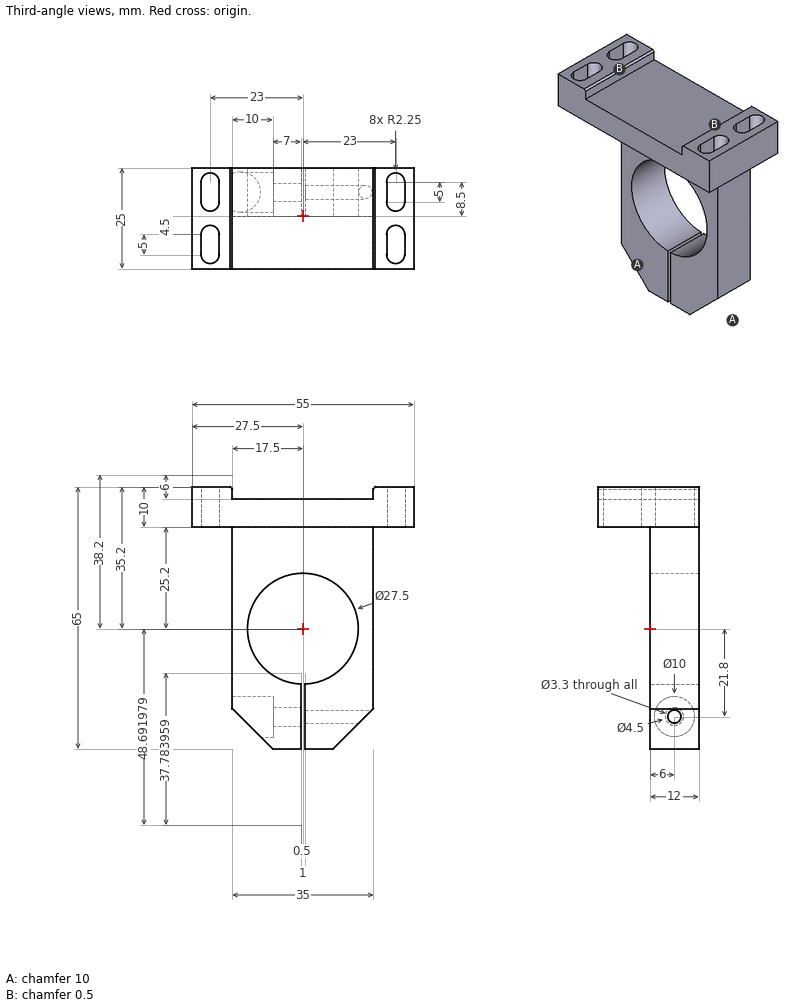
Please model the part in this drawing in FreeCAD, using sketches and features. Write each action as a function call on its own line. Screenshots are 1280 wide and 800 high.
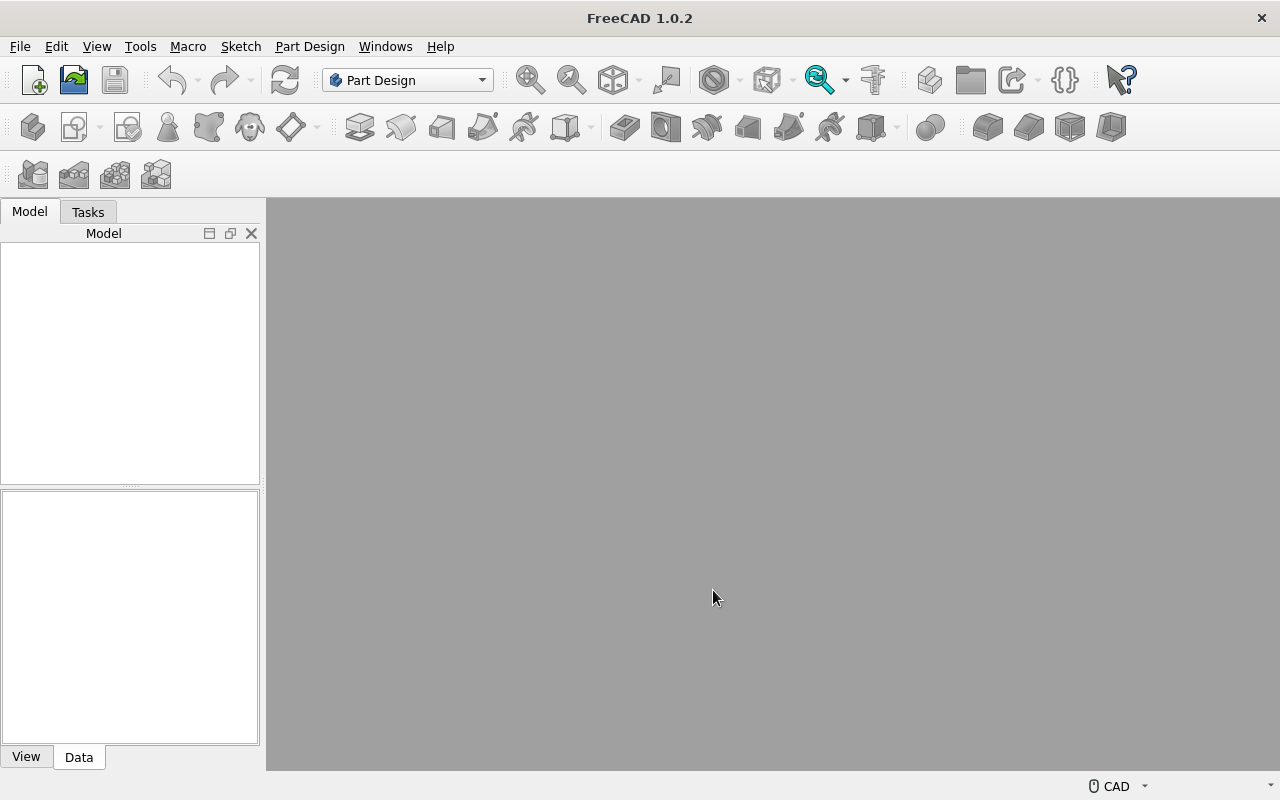
key(ctrl+n)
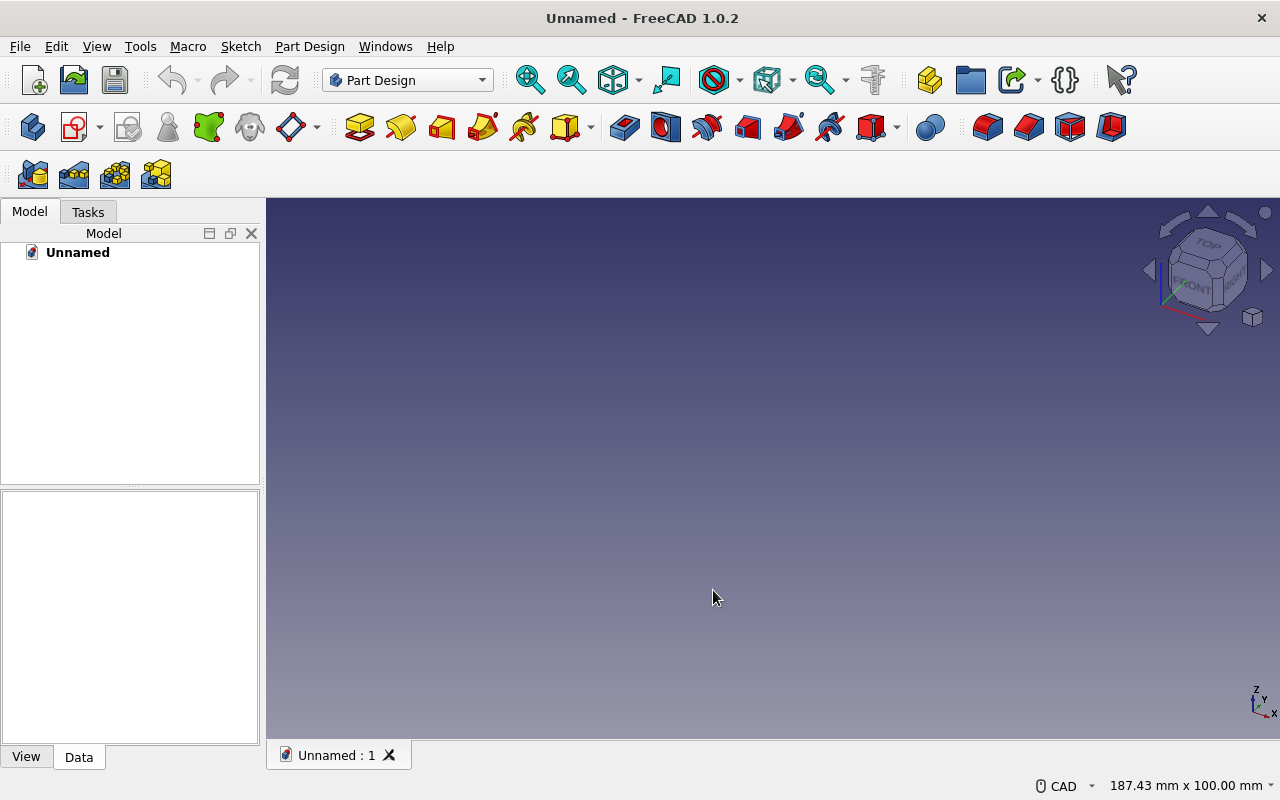
click(74, 128)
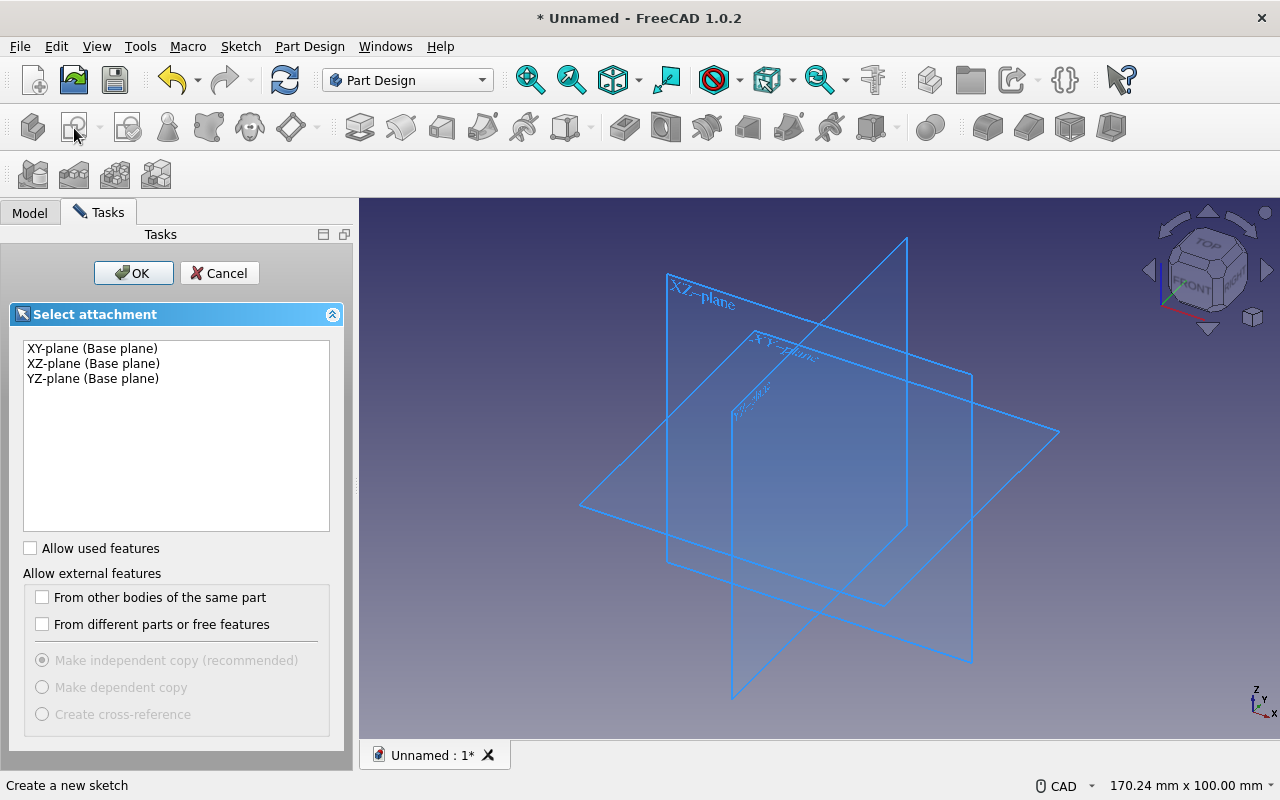
click(84, 364)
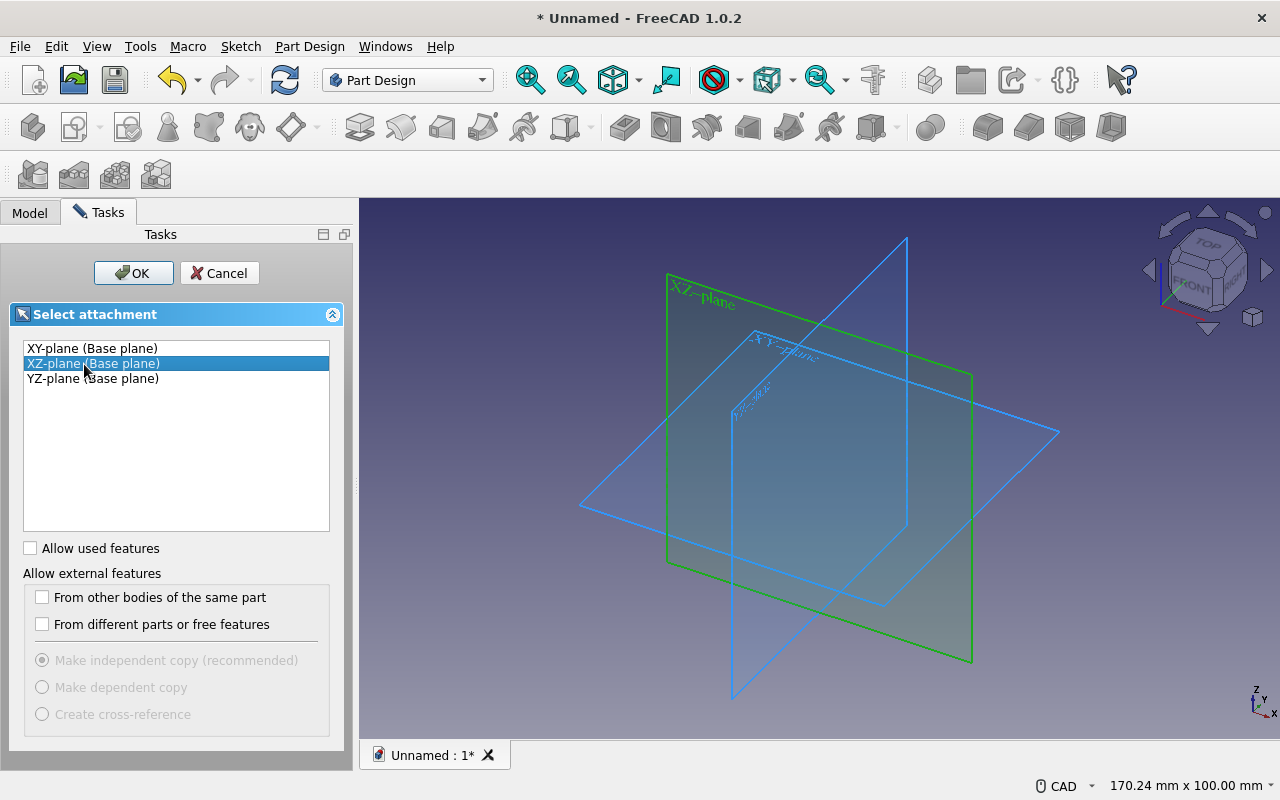
click(134, 273)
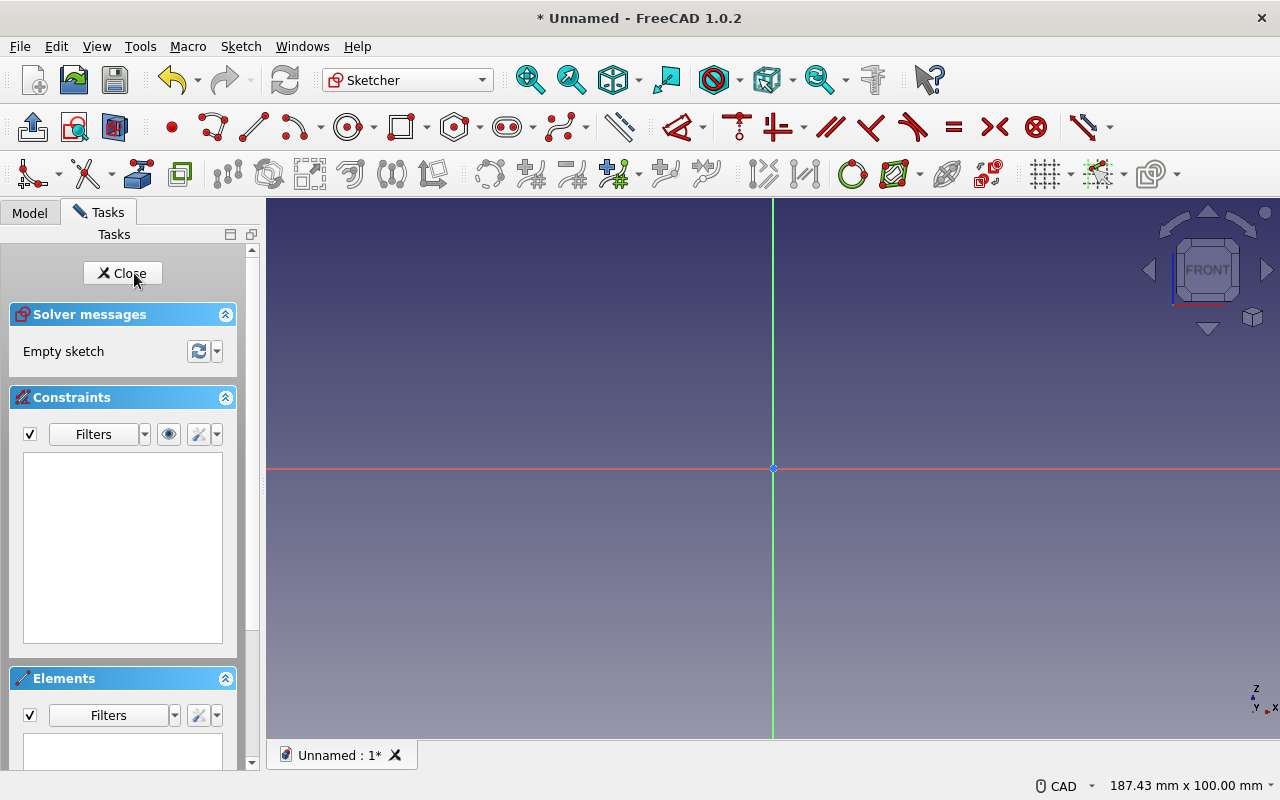
click(400, 128)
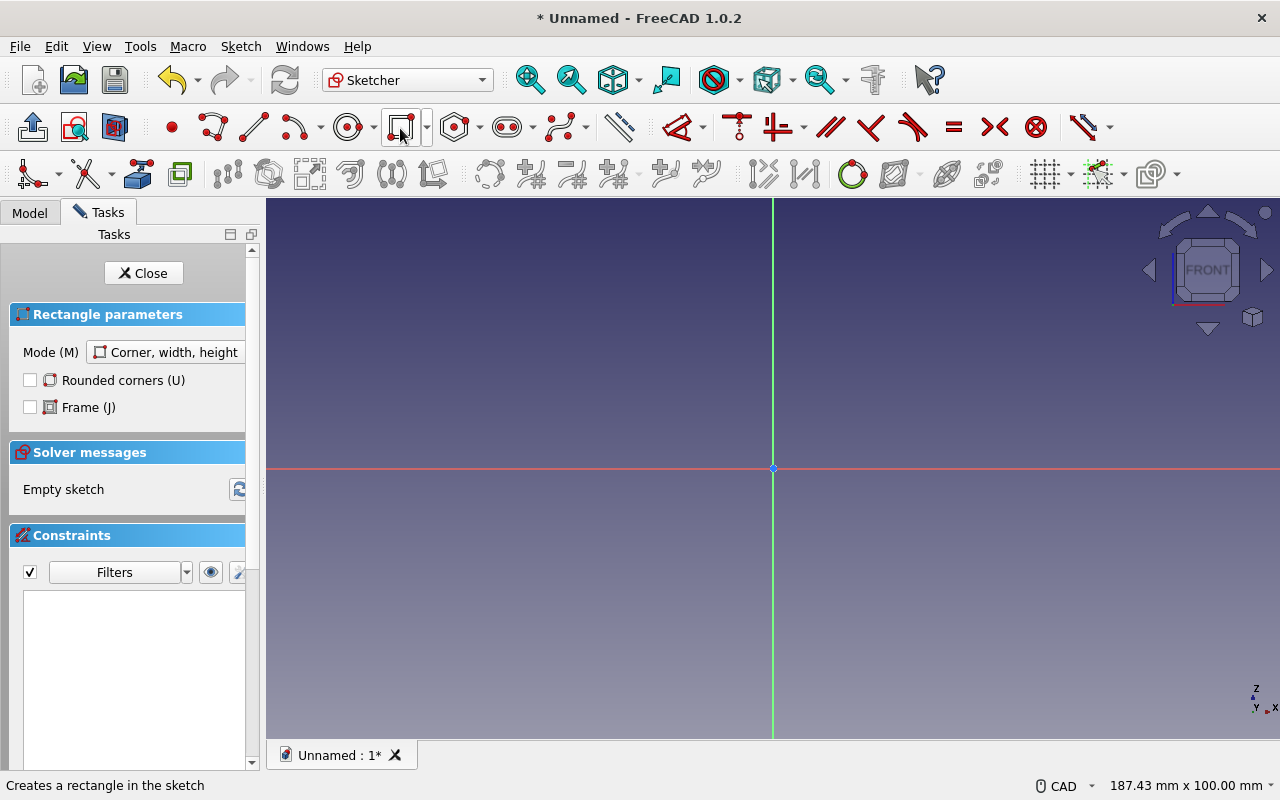
click(678, 278)
click(868, 630)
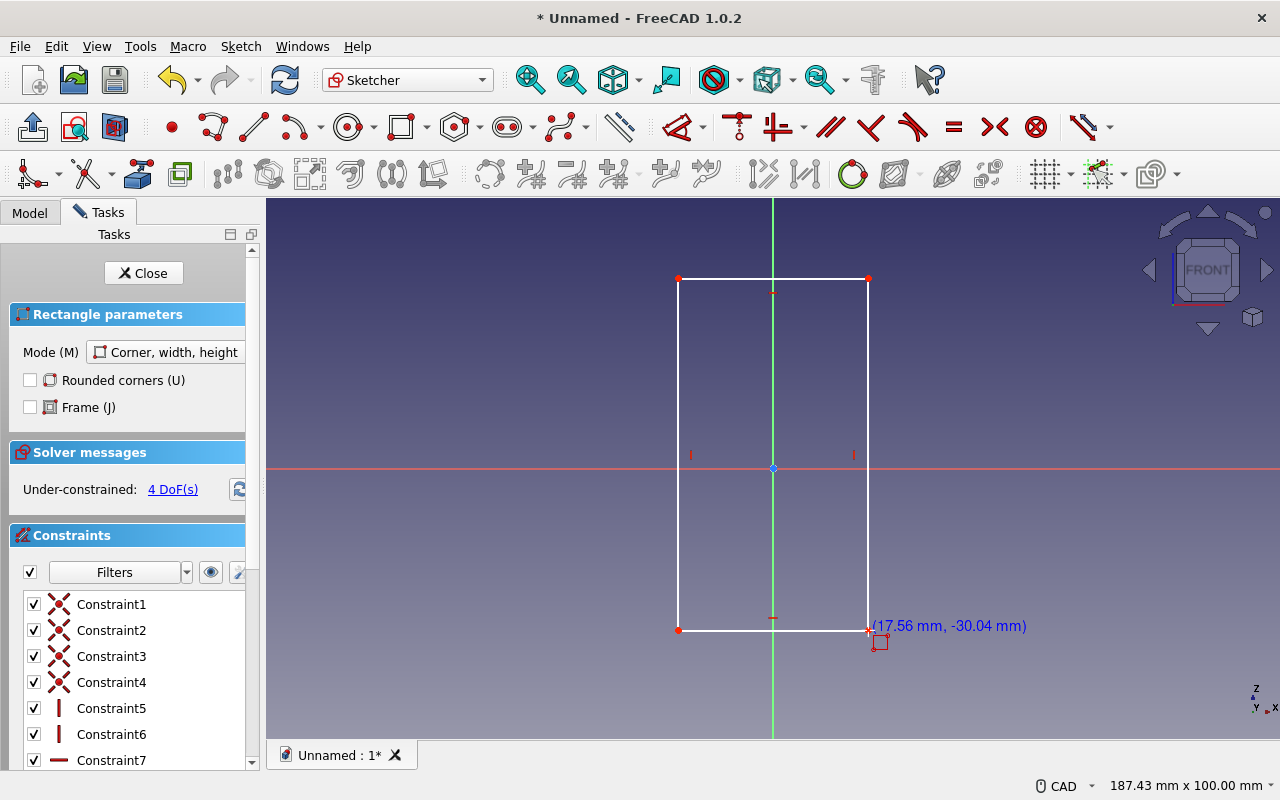
click(348, 128)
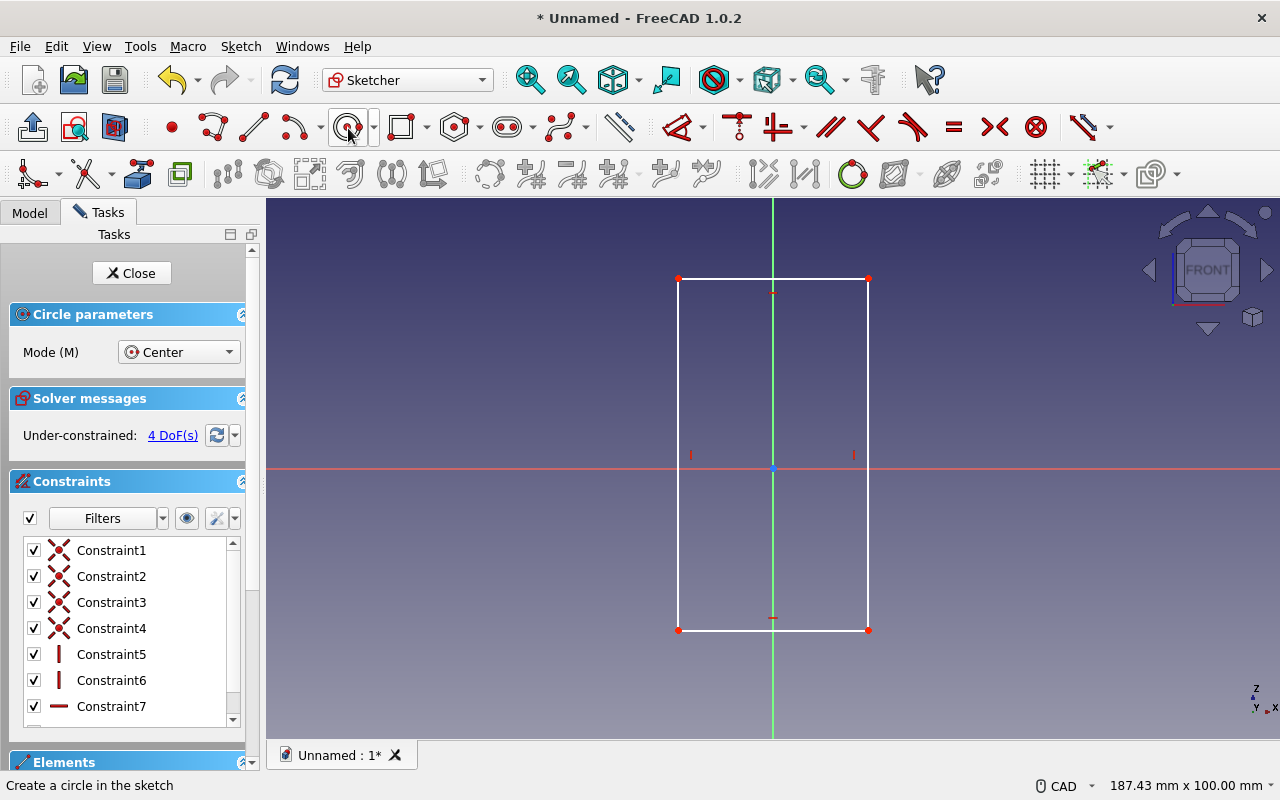
click(773, 468)
click(826, 416)
key(Escape)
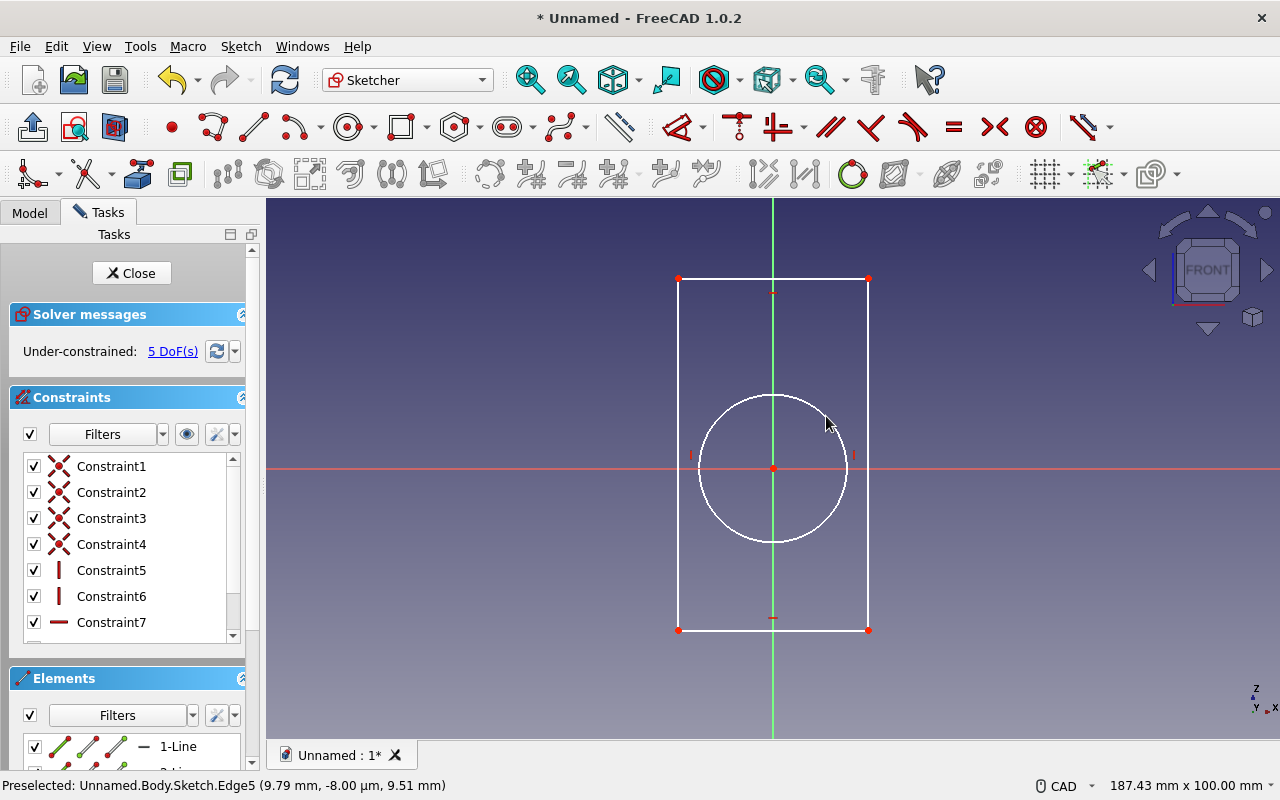
click(676, 128)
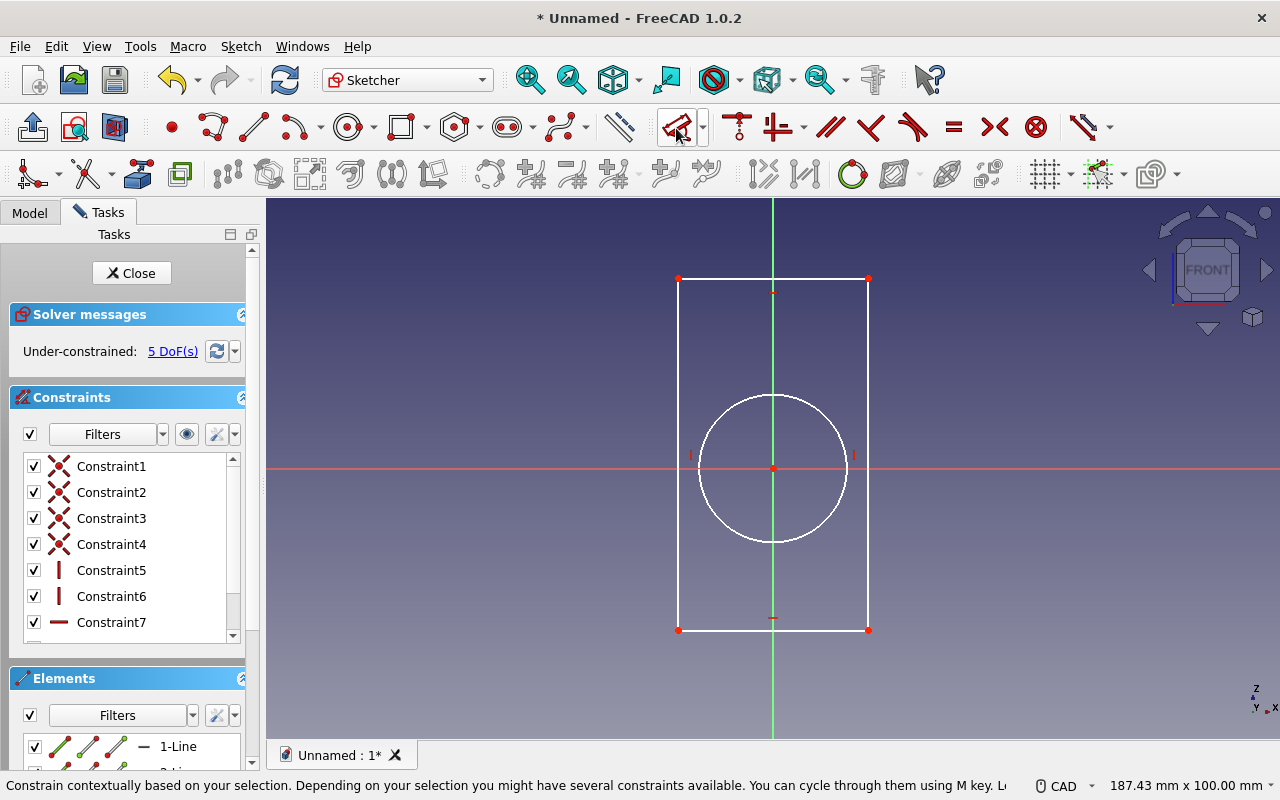
click(825, 416)
click(848, 393)